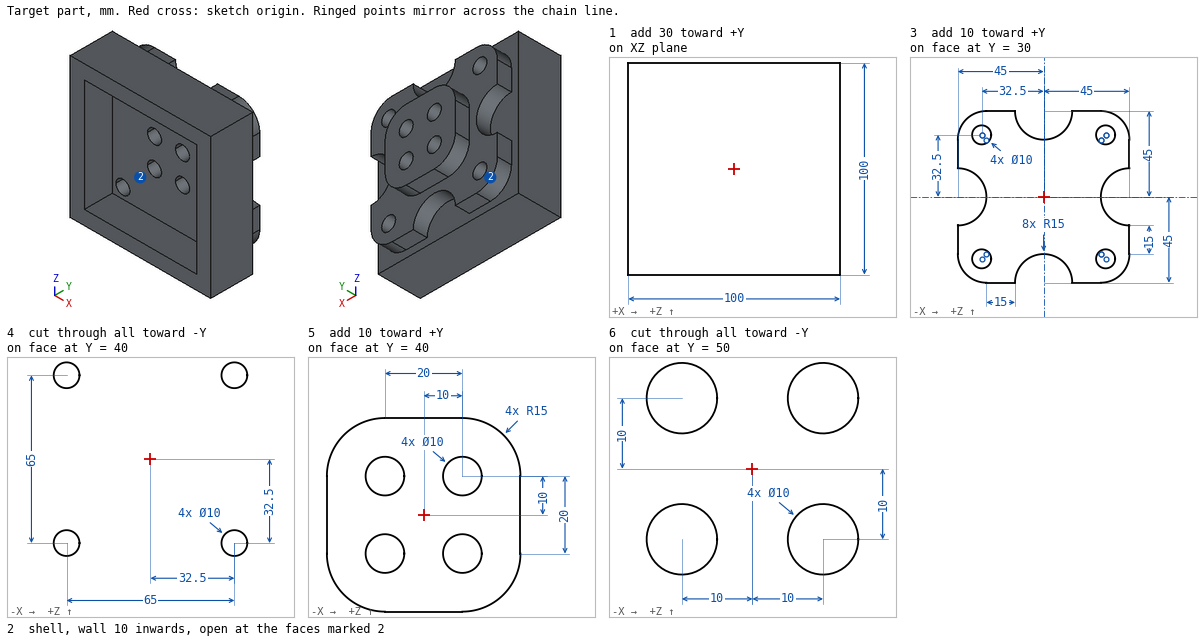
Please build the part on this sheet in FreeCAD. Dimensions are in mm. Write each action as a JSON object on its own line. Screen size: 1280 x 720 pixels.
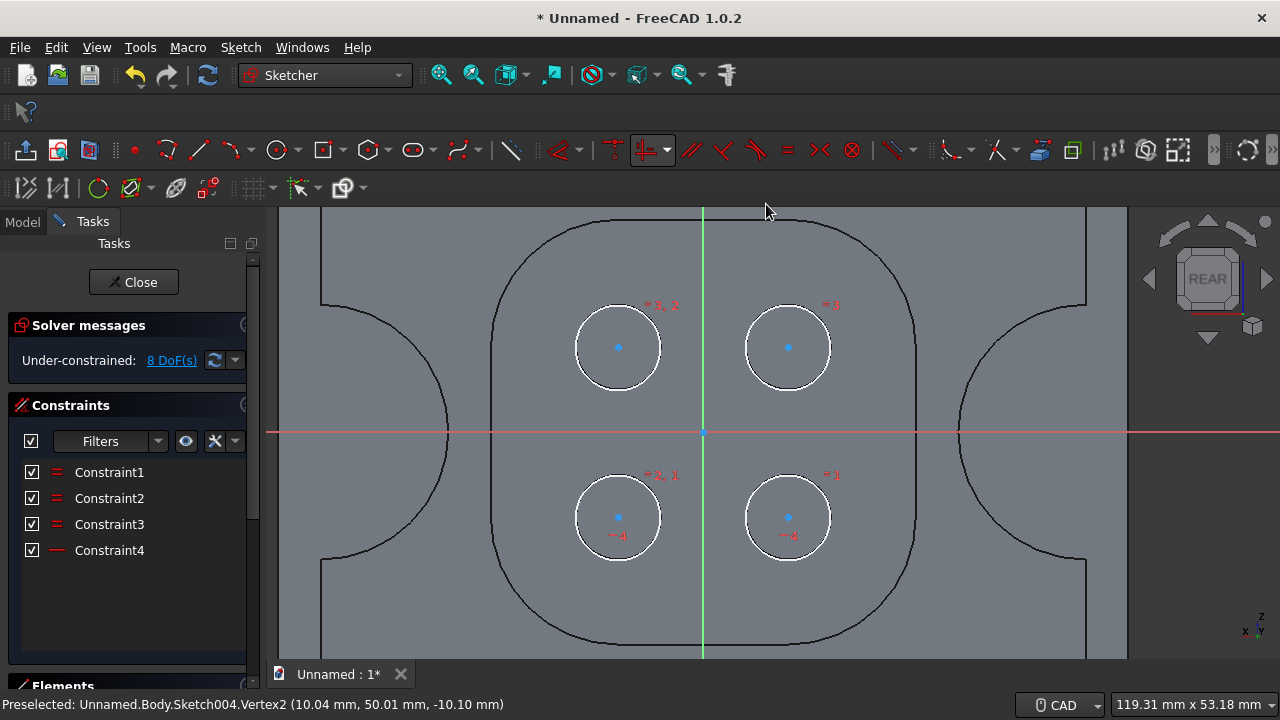
{"action": "left_click", "coordinate": [618, 518]}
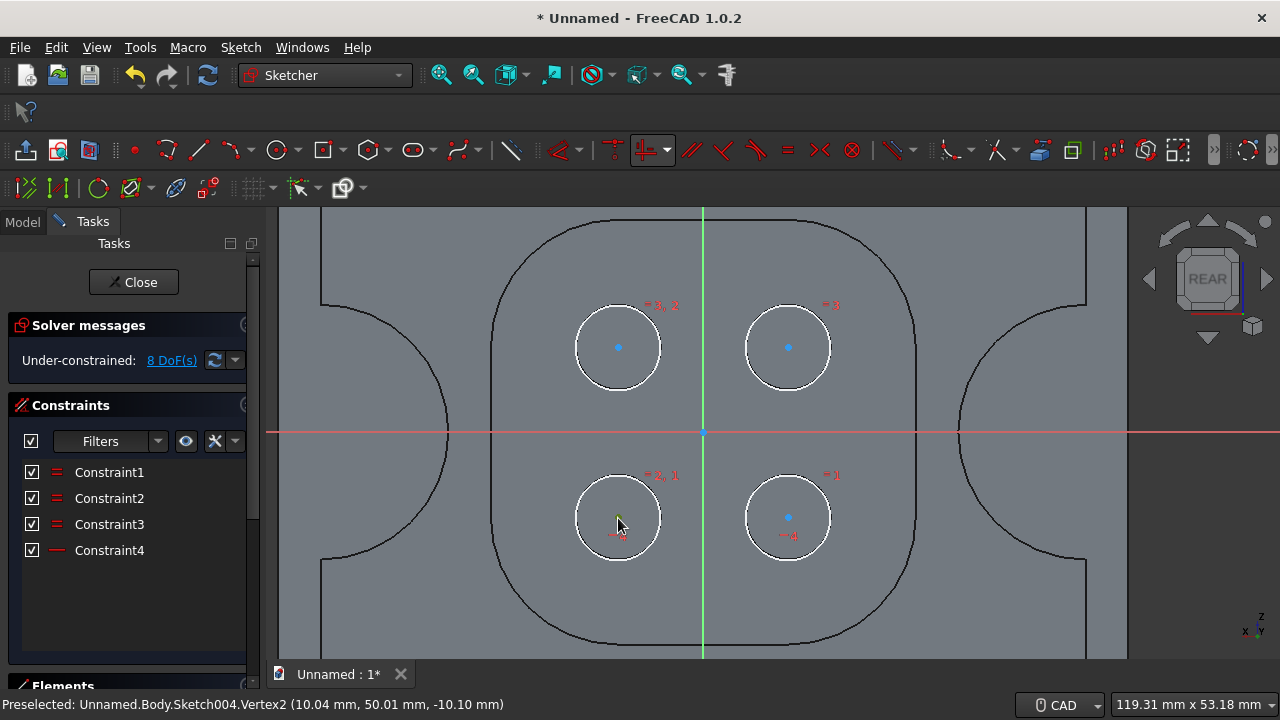
{"action": "left_click", "coordinate": [618, 348]}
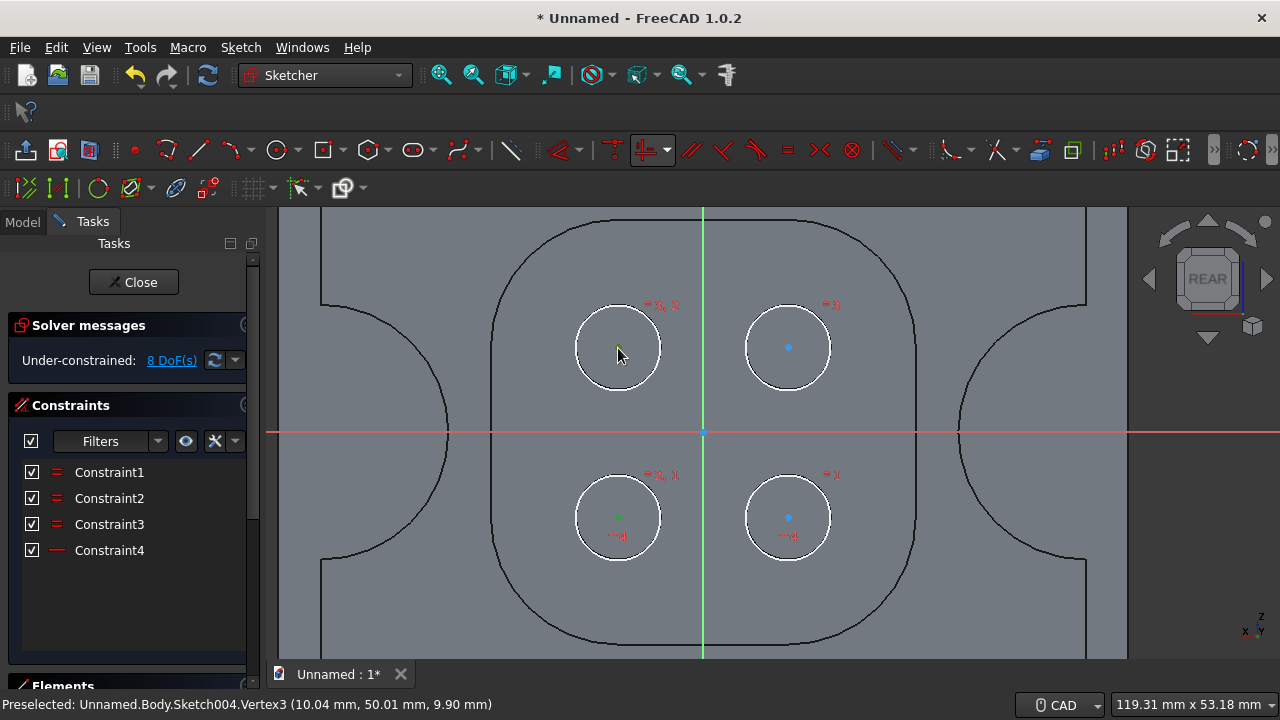
{"action": "left_click", "coordinate": [670, 150]}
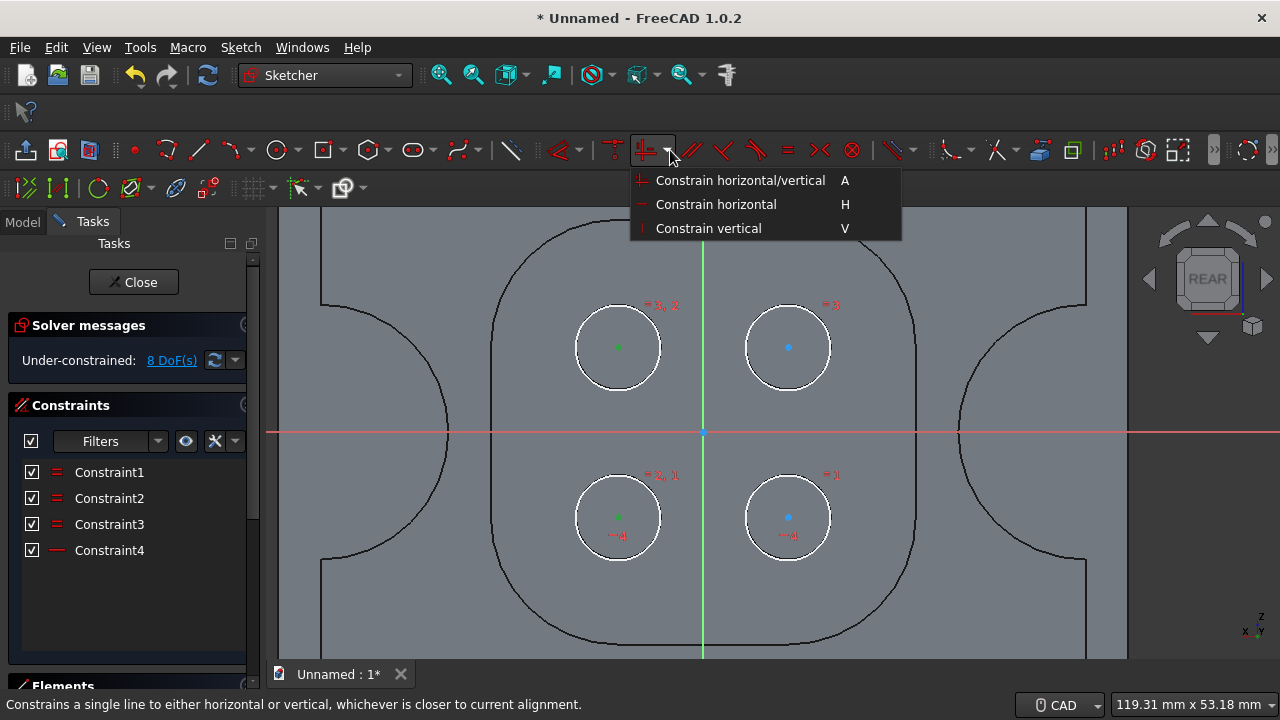
{"action": "left_click", "coordinate": [766, 228]}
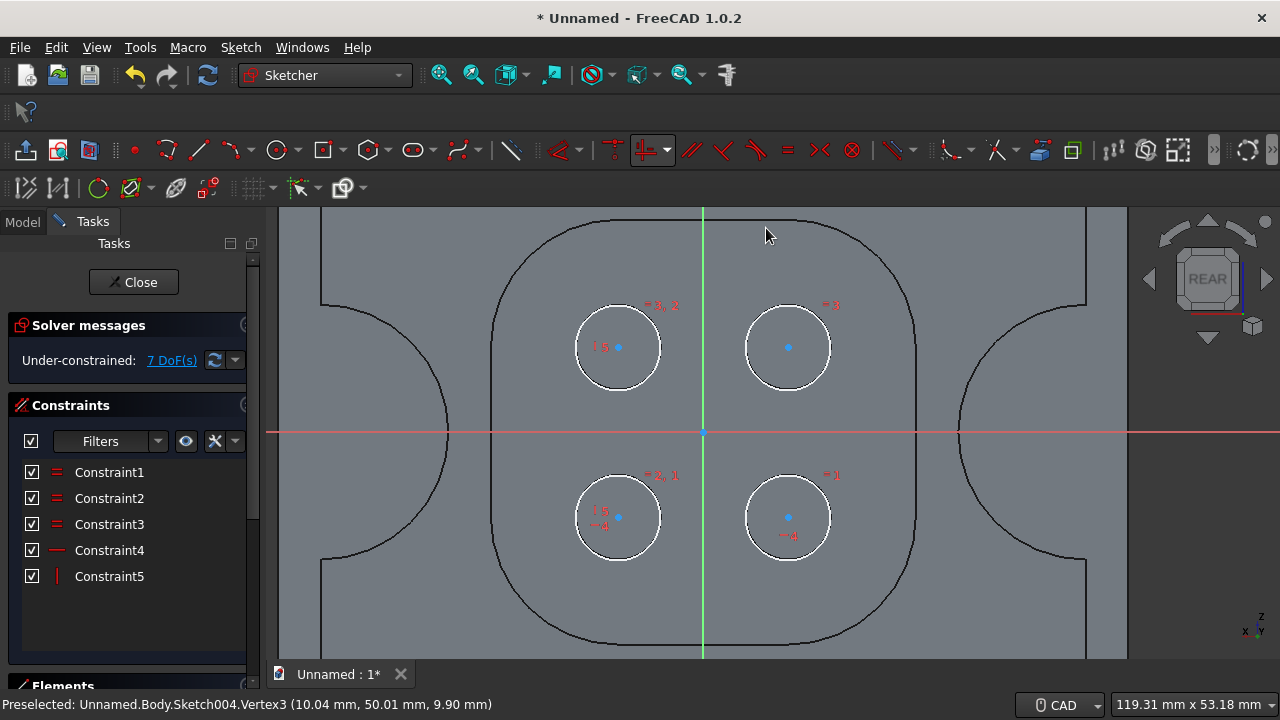
{"action": "left_click", "coordinate": [788, 518]}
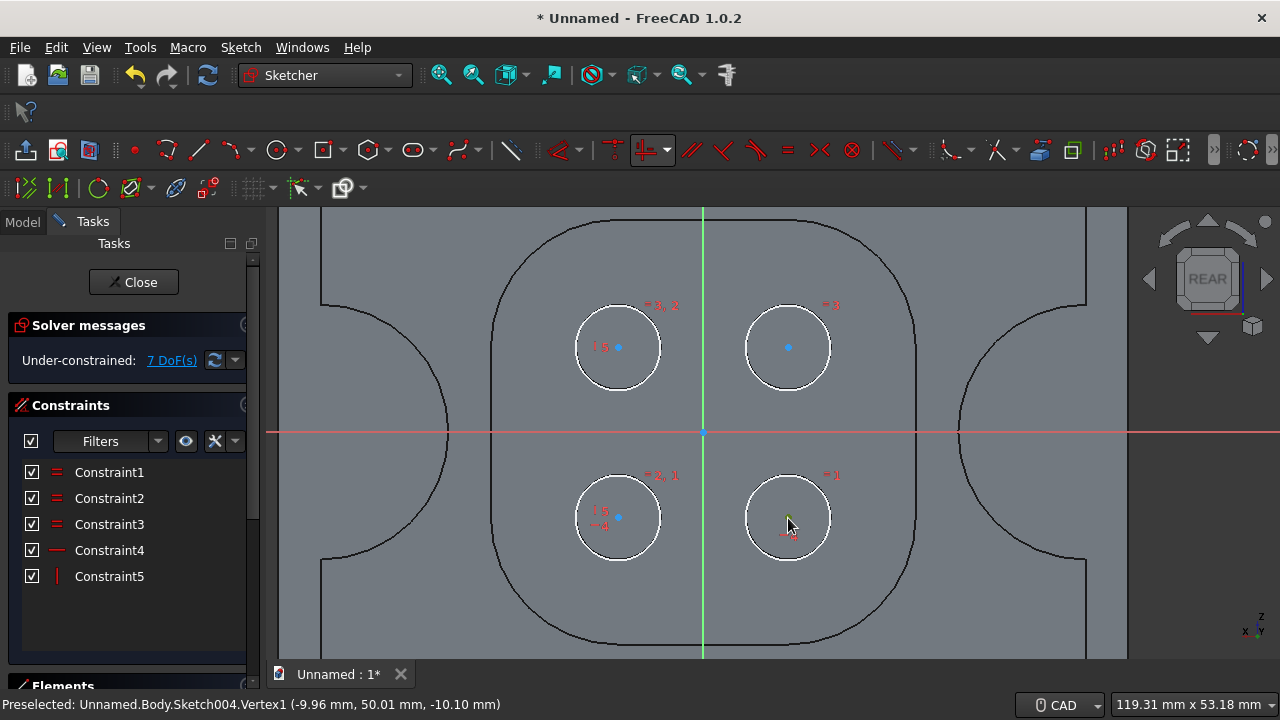
{"action": "left_click", "coordinate": [788, 348]}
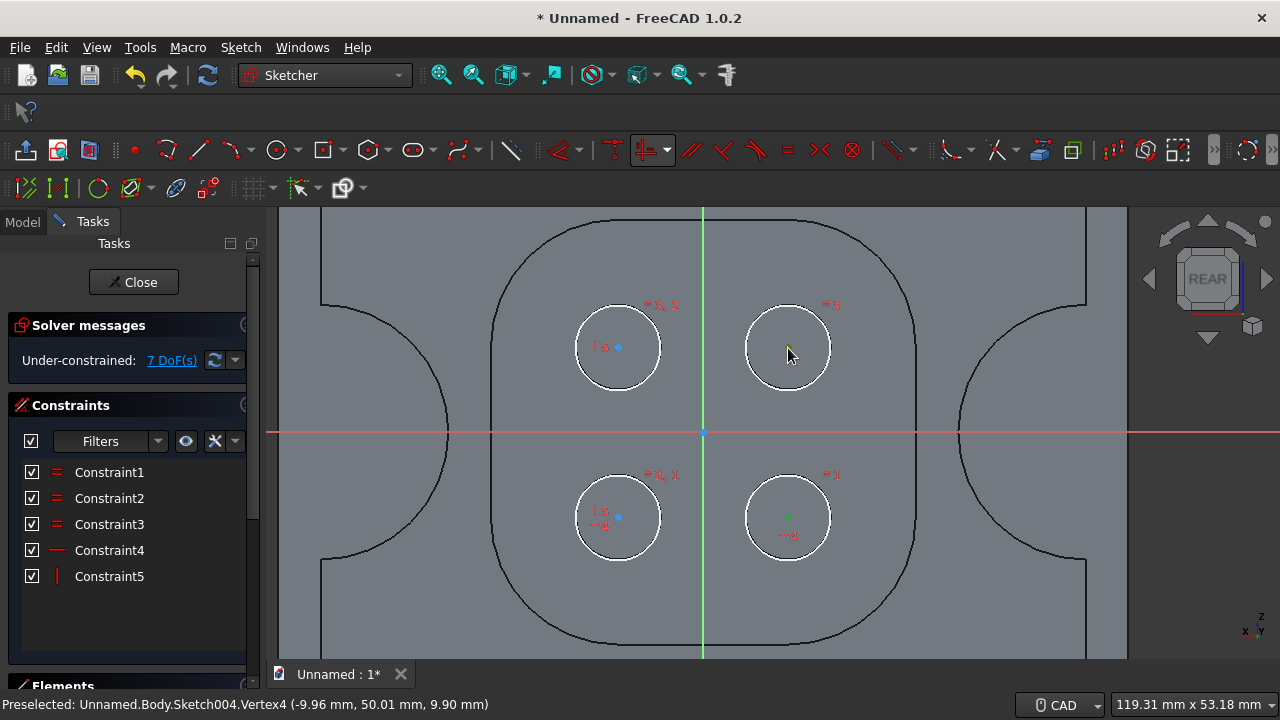
{"action": "left_click", "coordinate": [670, 150]}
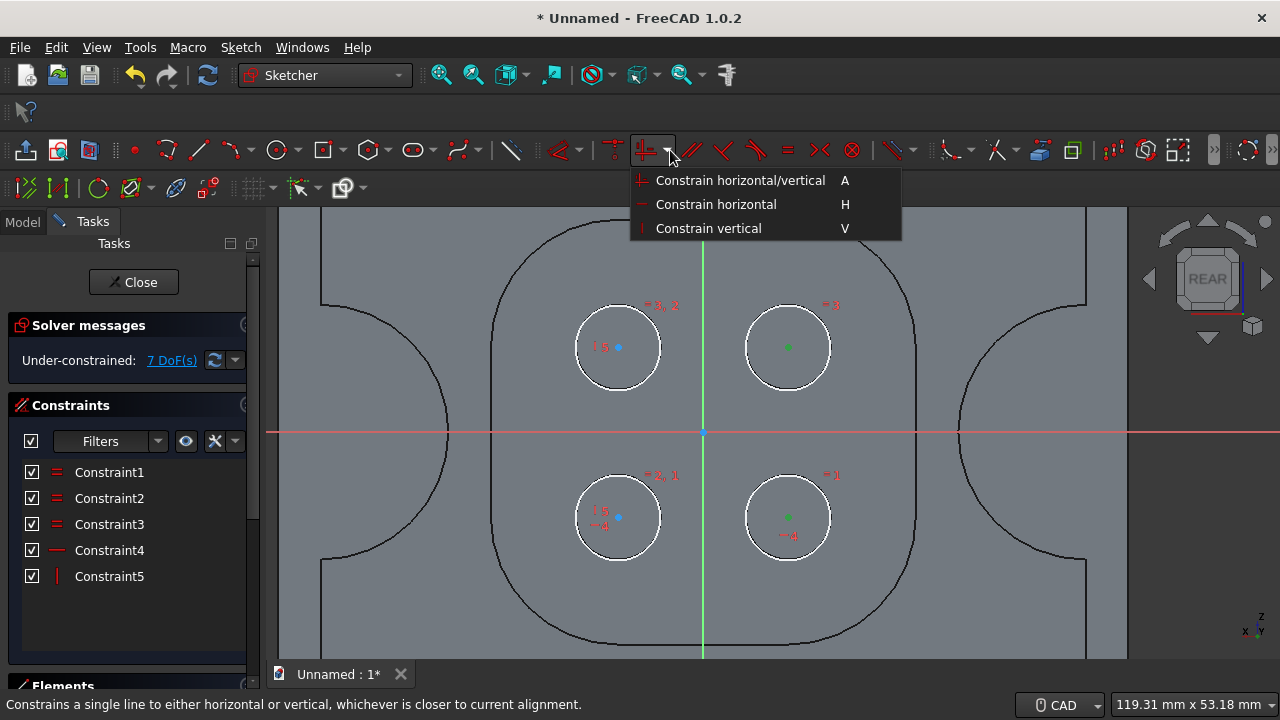
{"action": "left_click", "coordinate": [766, 228]}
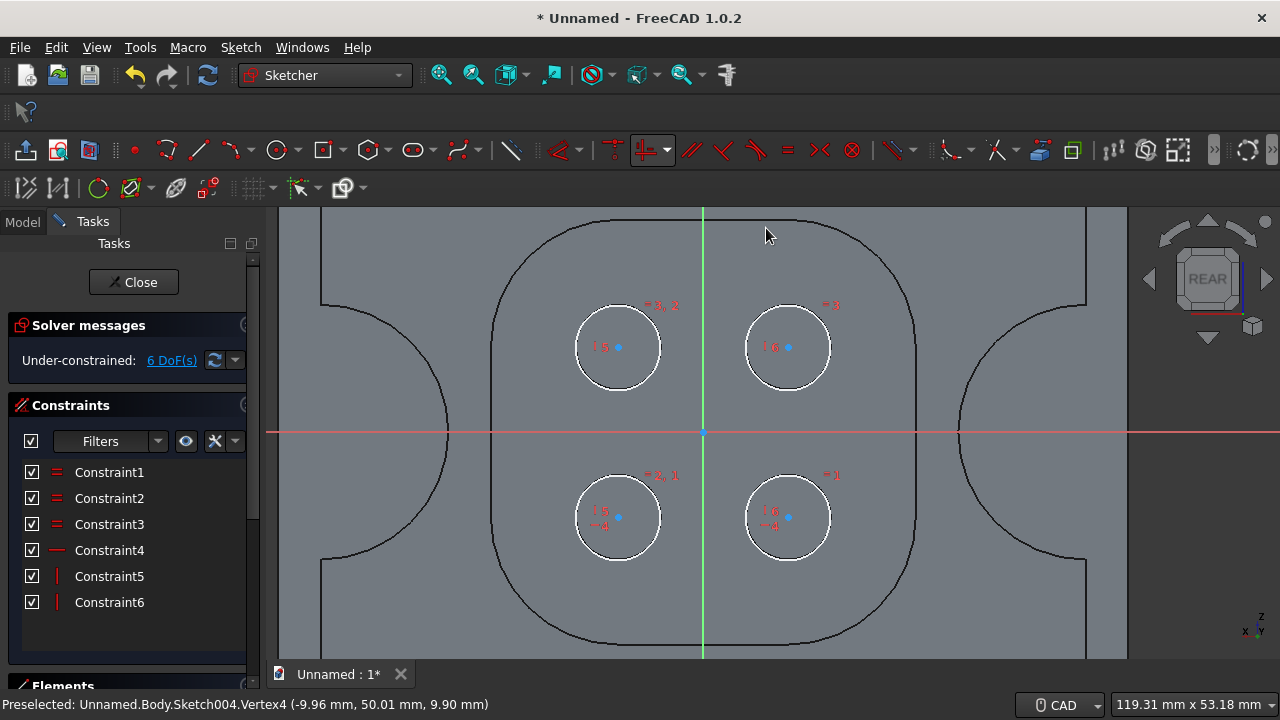
{"action": "left_click", "coordinate": [618, 348]}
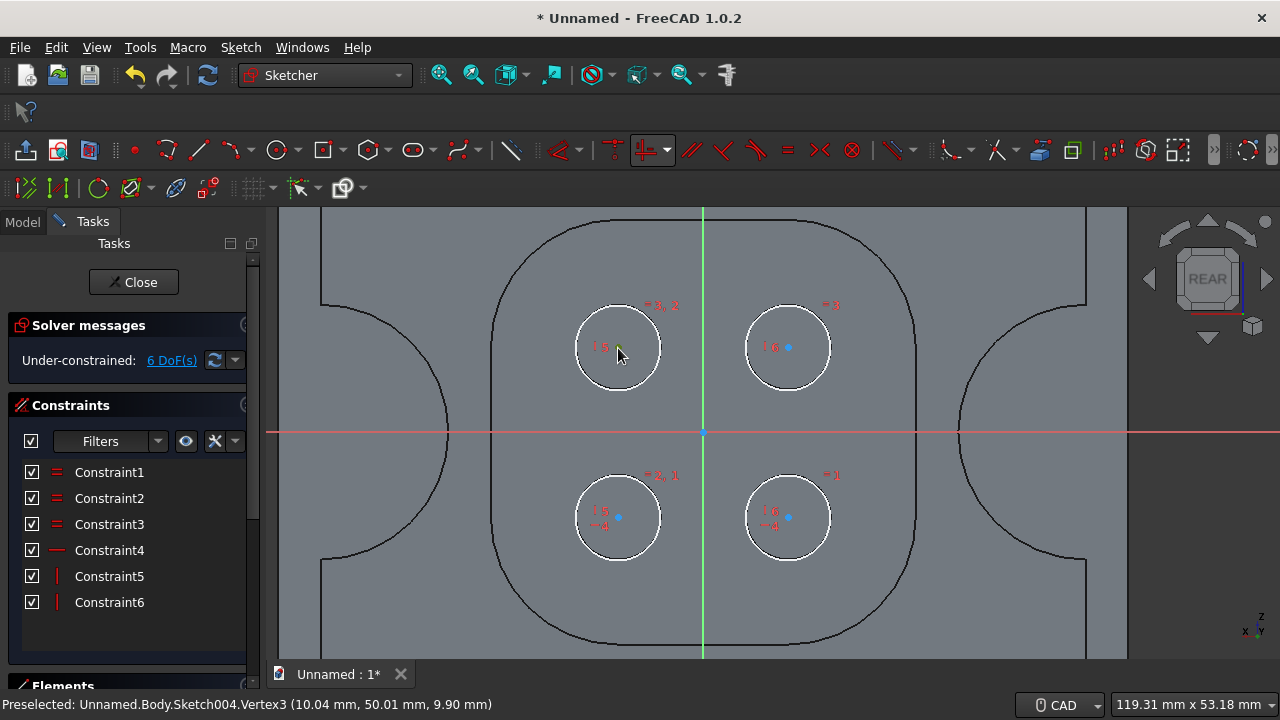
{"action": "left_click", "coordinate": [788, 348]}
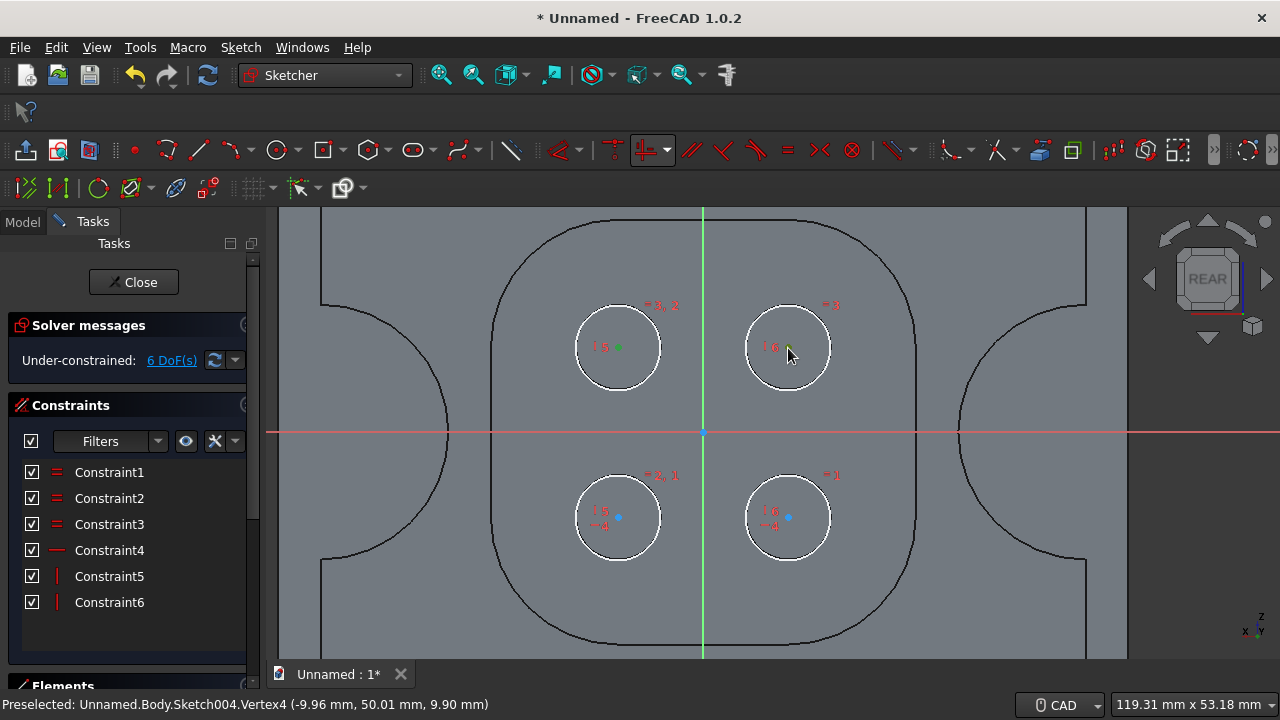
{"action": "left_click", "coordinate": [670, 150]}